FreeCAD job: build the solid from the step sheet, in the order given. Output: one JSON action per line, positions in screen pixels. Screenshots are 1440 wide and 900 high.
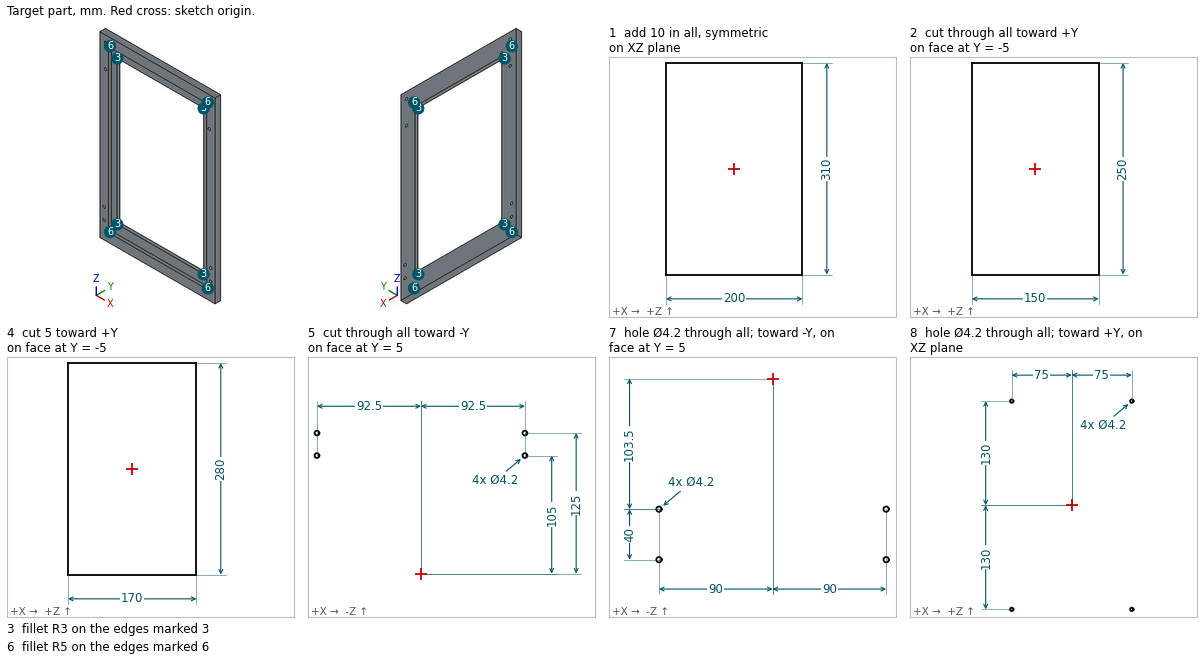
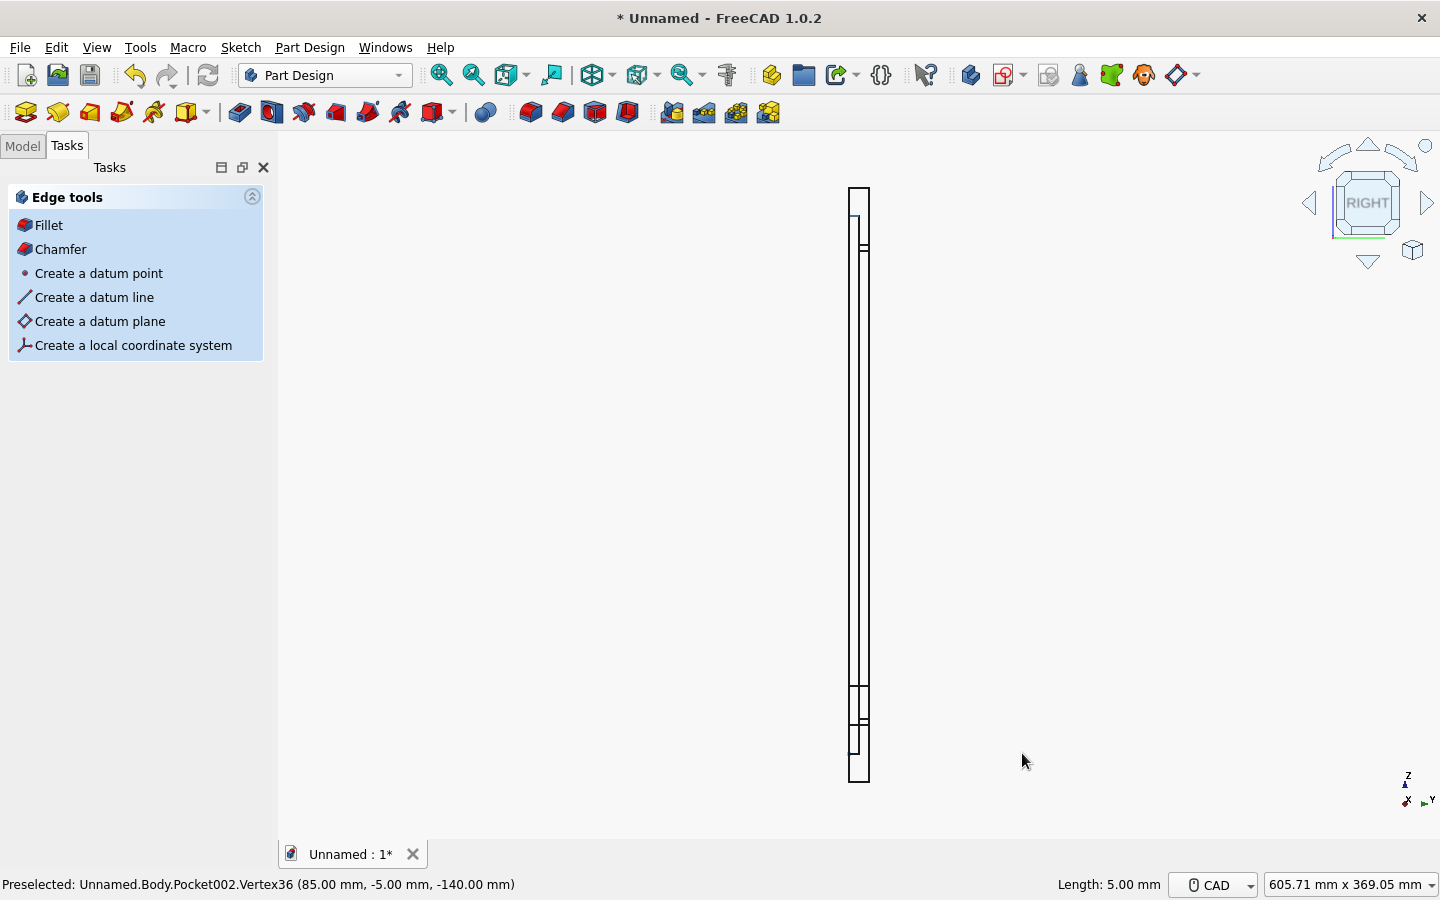
{"action": "scroll", "coordinate": [854, 753], "scroll_direction": "up", "scroll_amount": 8}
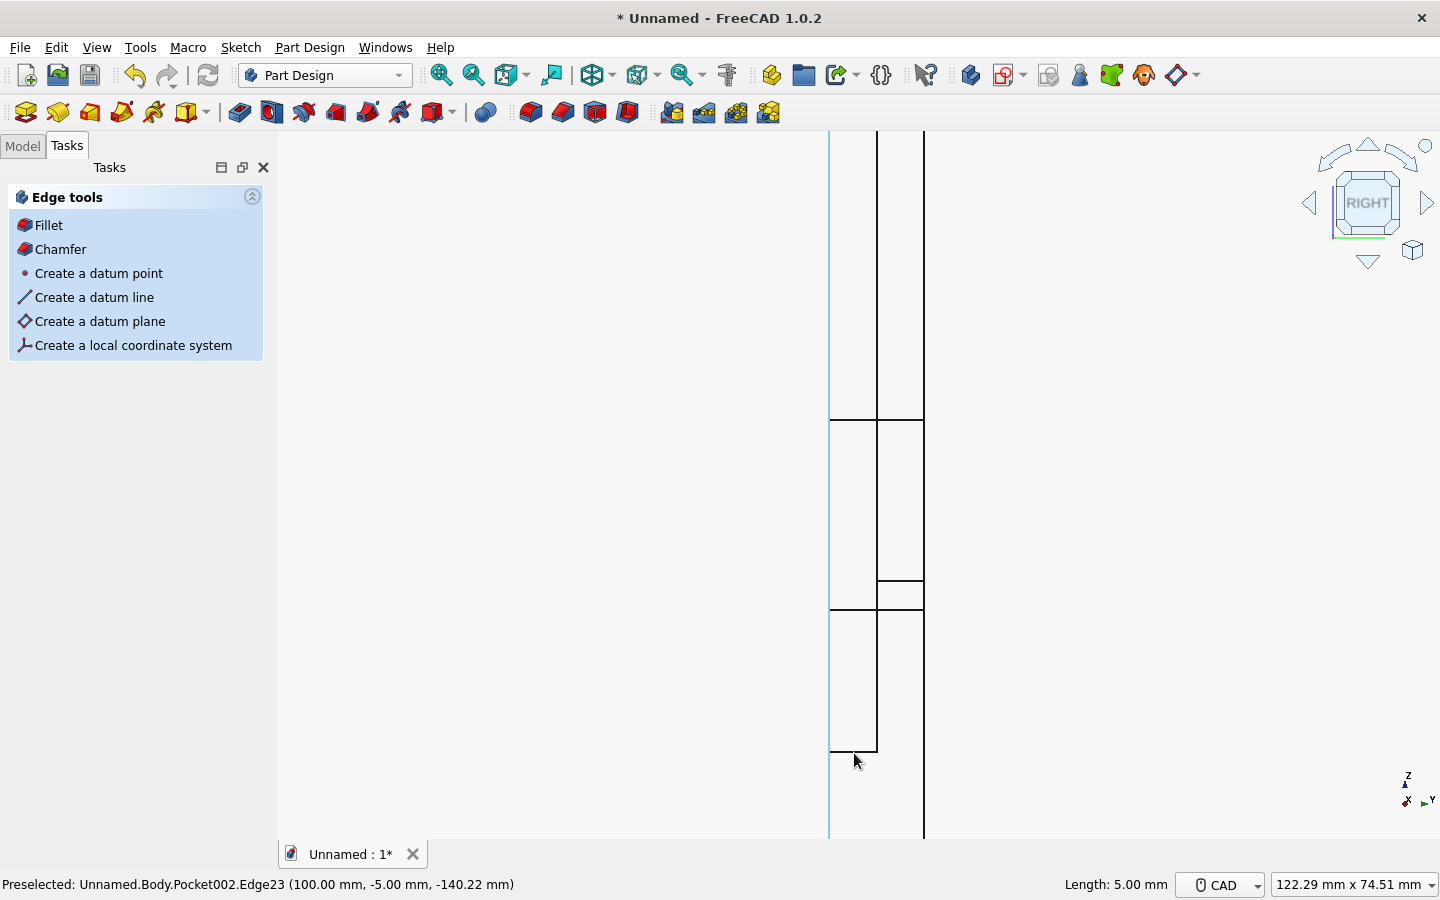
{"action": "left_click", "coordinate": [853, 751], "text": "ctrl"}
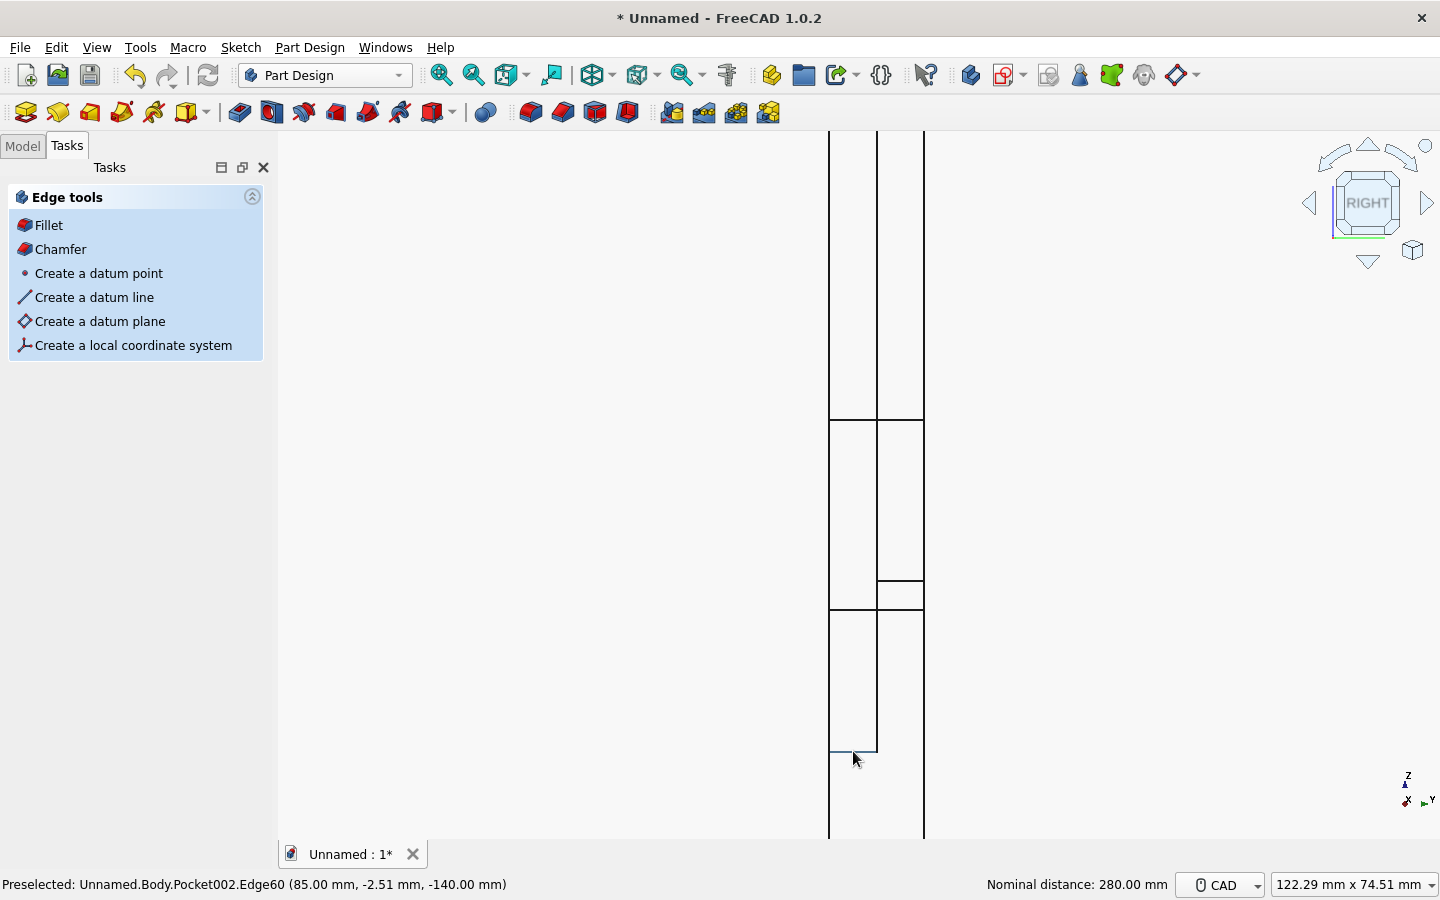
{"action": "key", "text": "v f"}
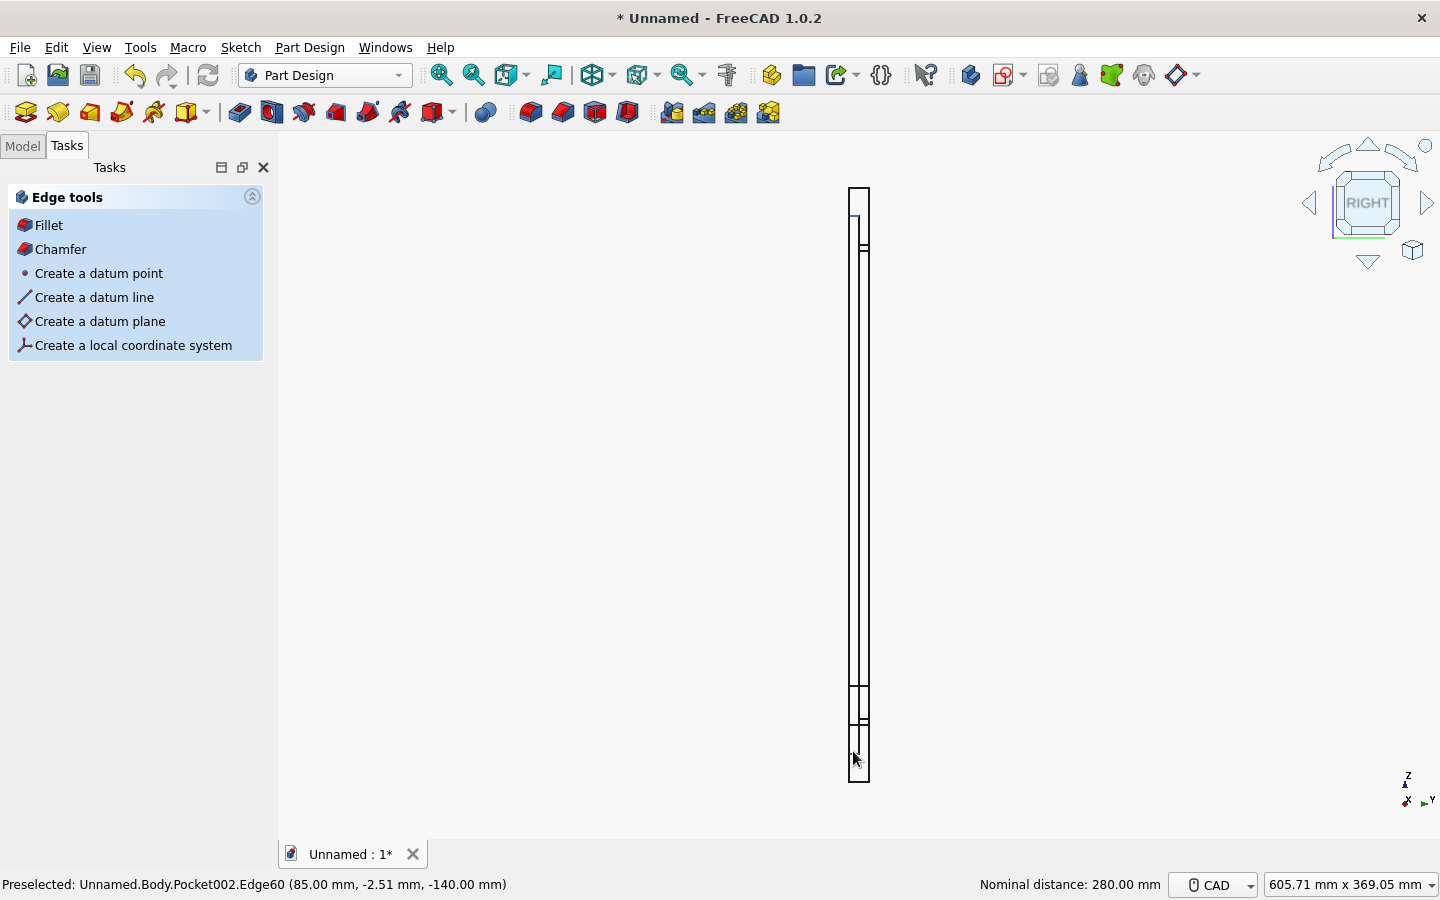
{"action": "key", "text": "5"}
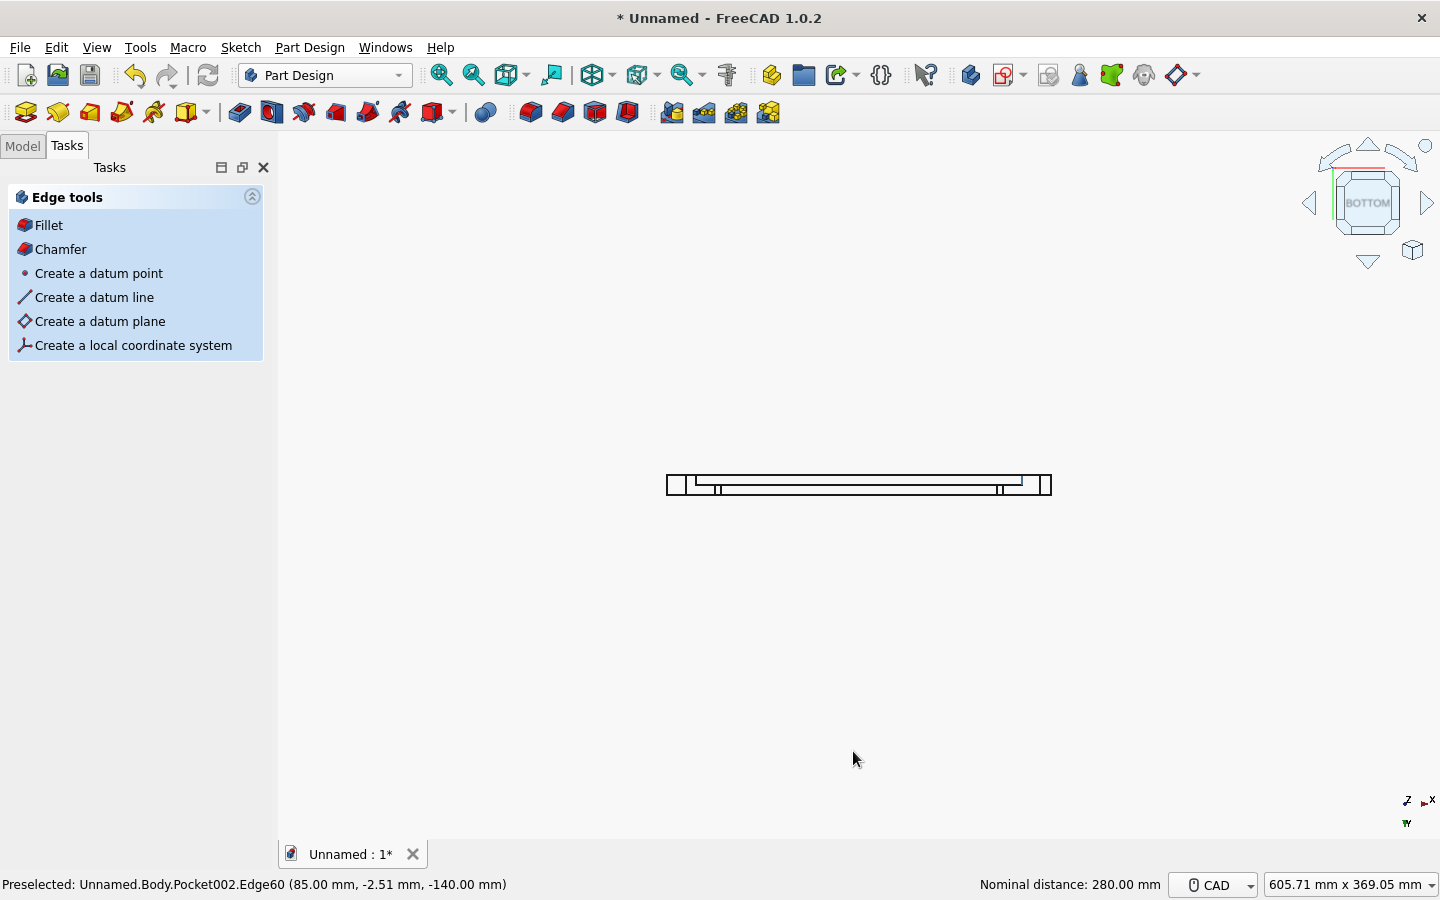
{"action": "key", "text": "v f"}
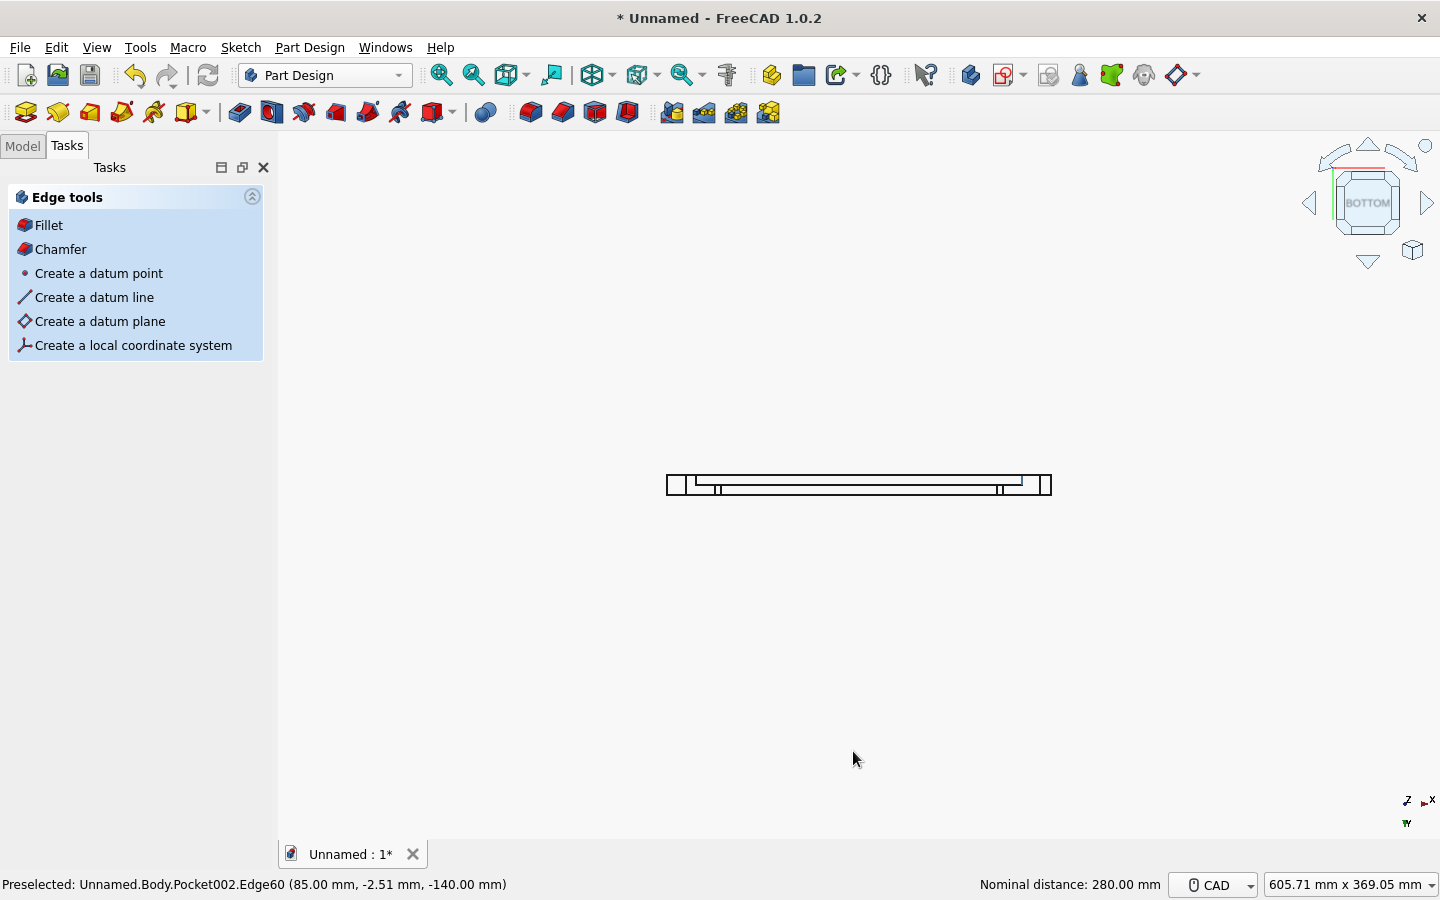
{"action": "left_click", "coordinate": [696, 481], "text": "ctrl"}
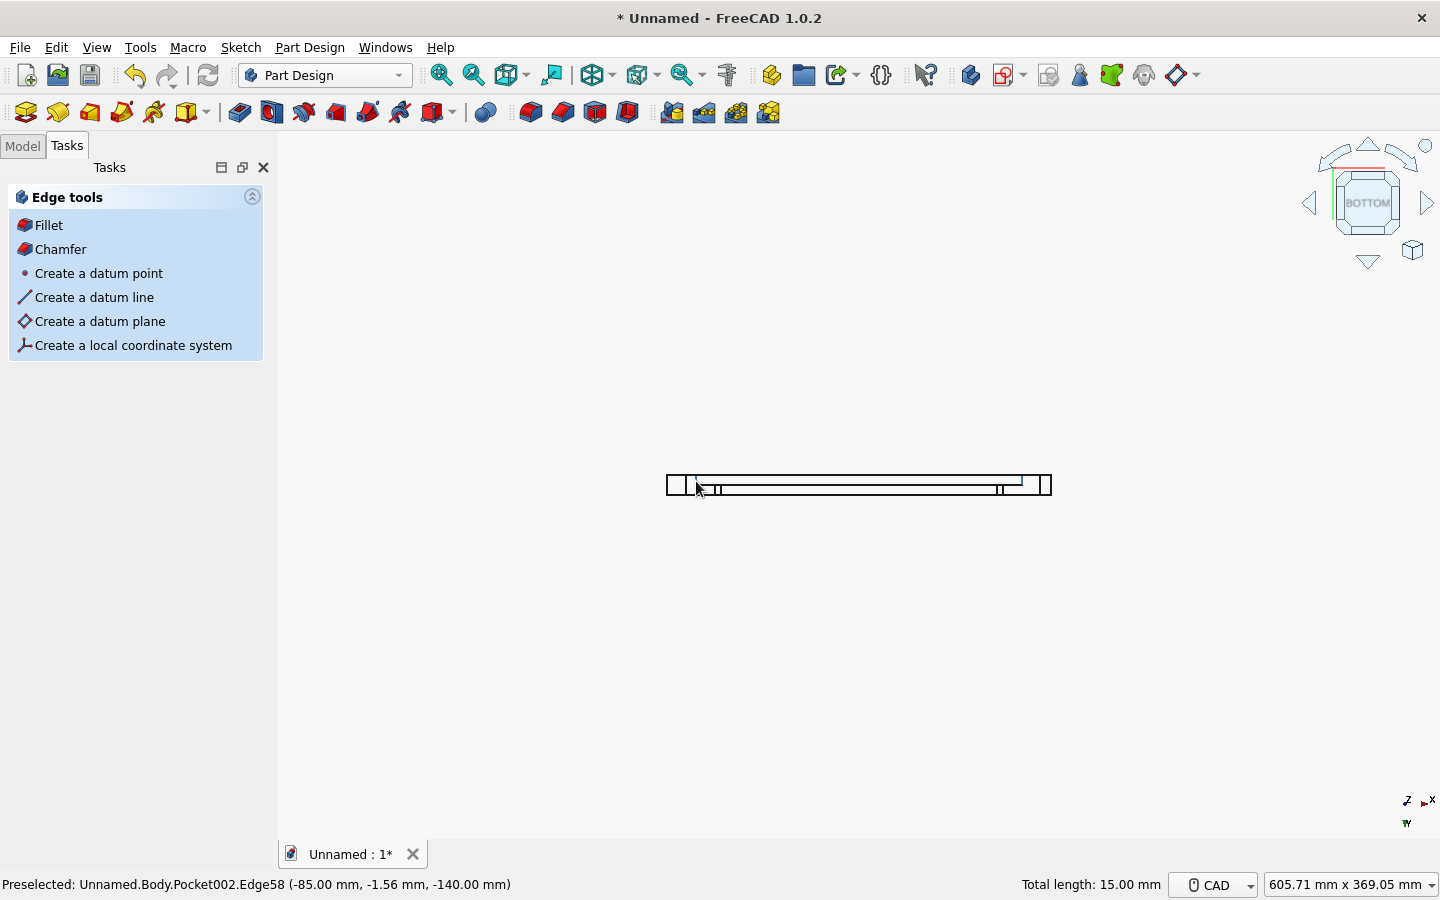
{"action": "scroll", "coordinate": [696, 479], "scroll_direction": "up", "scroll_amount": 8}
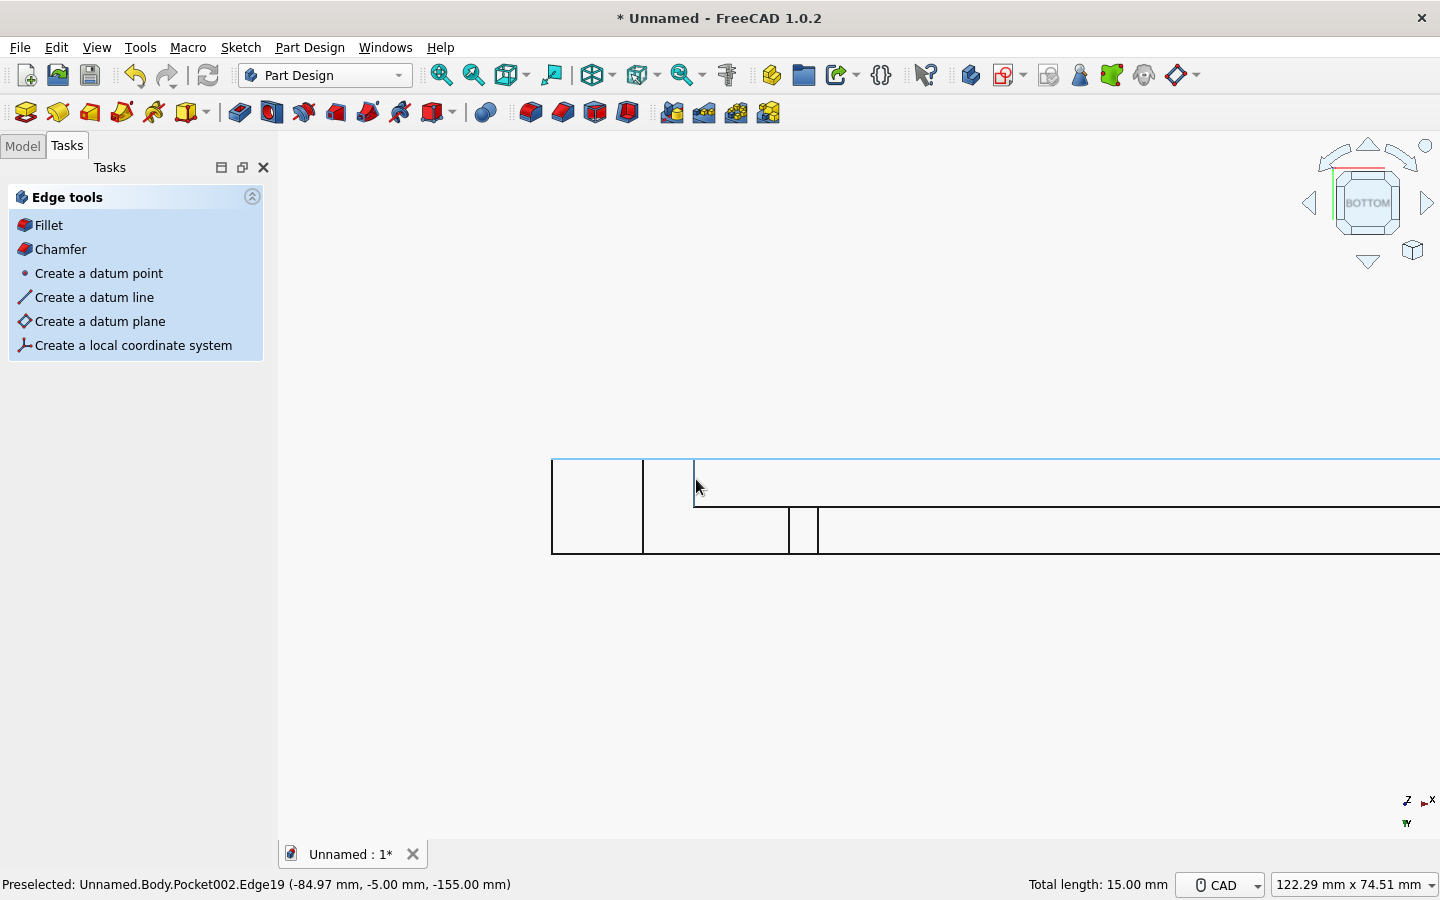
{"action": "key", "text": "v f"}